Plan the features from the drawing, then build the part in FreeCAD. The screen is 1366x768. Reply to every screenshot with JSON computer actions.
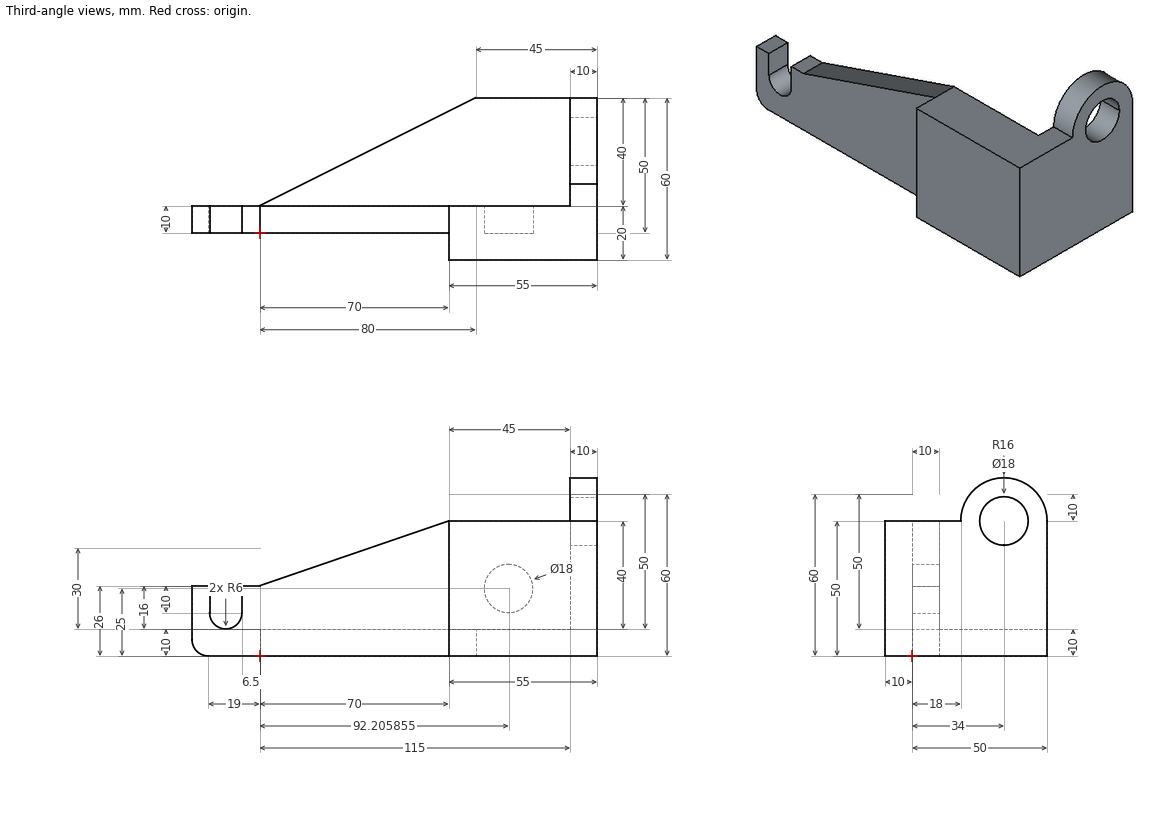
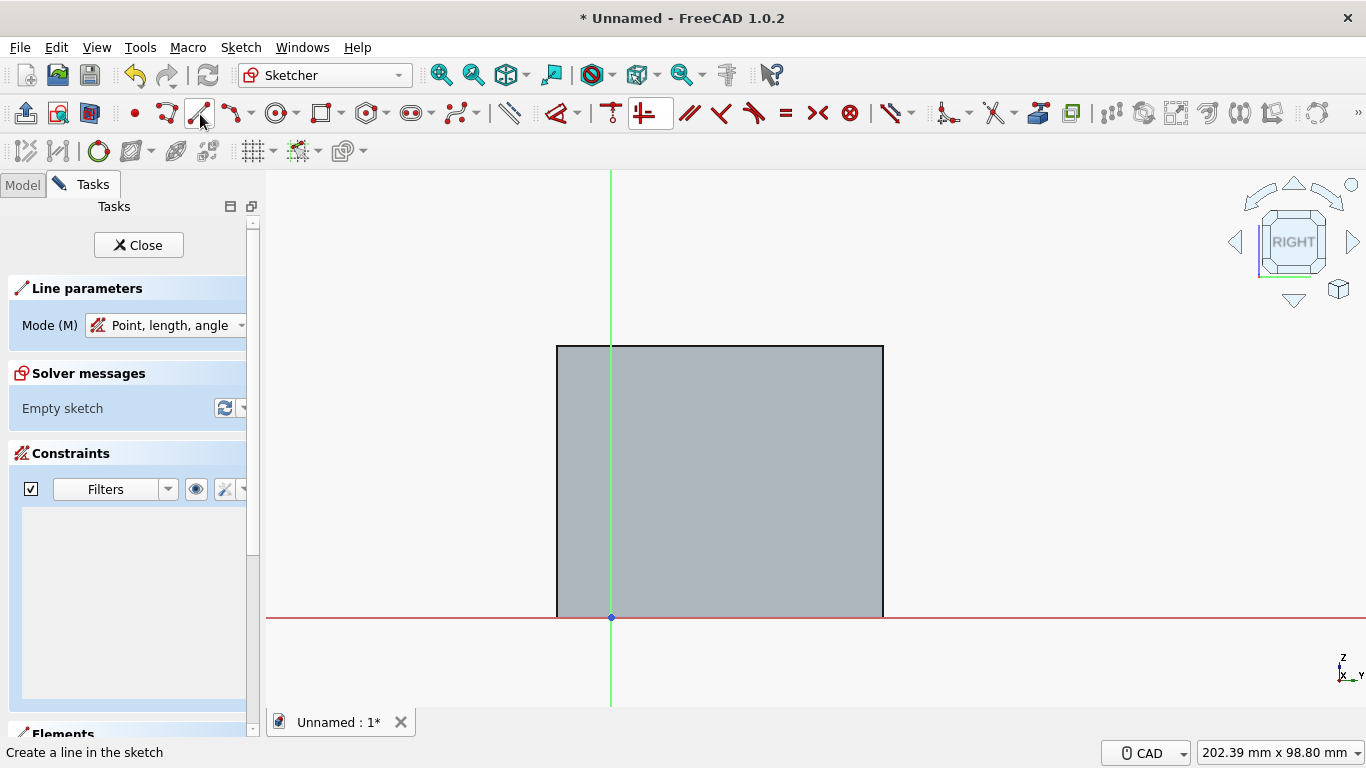
{"action": "left_click", "coordinate": [709, 346]}
{"action": "left_click", "coordinate": [883, 346]}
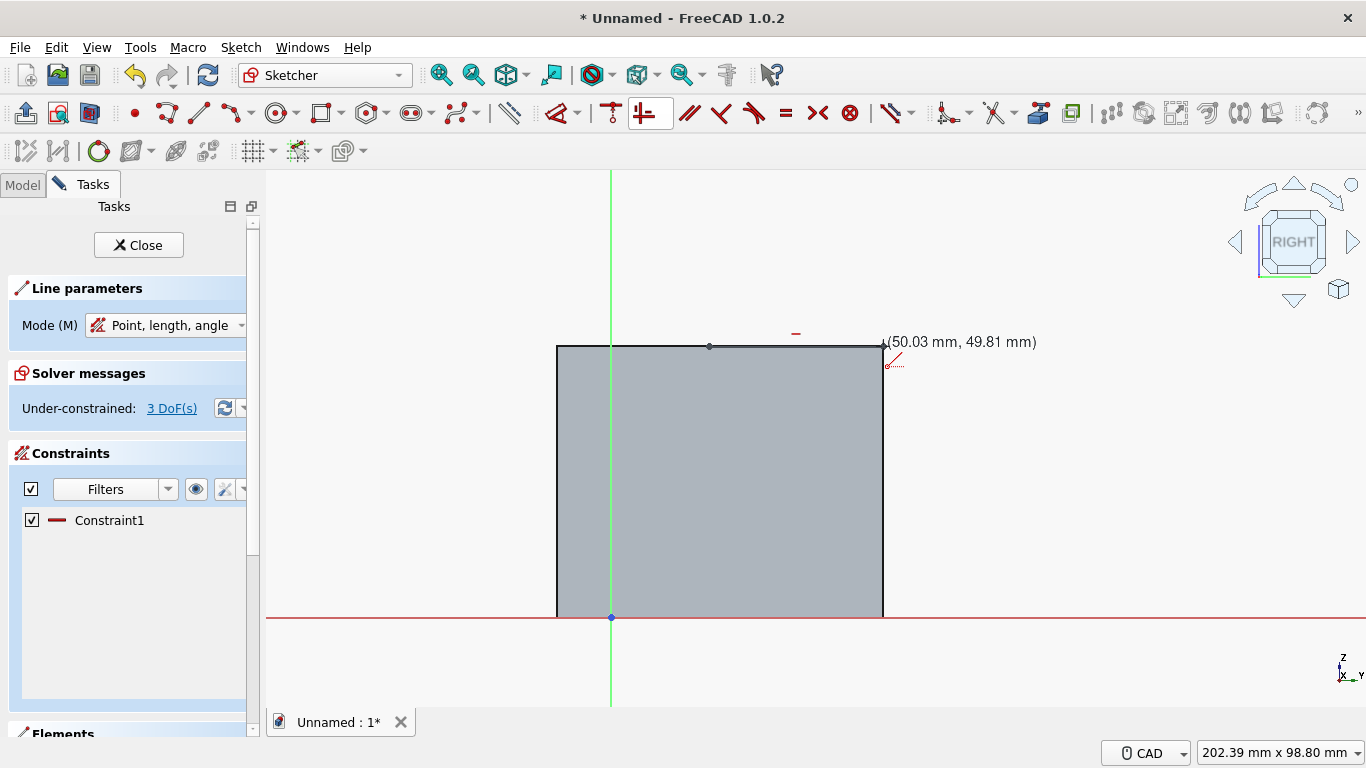
{"action": "left_click", "coordinate": [232, 114]}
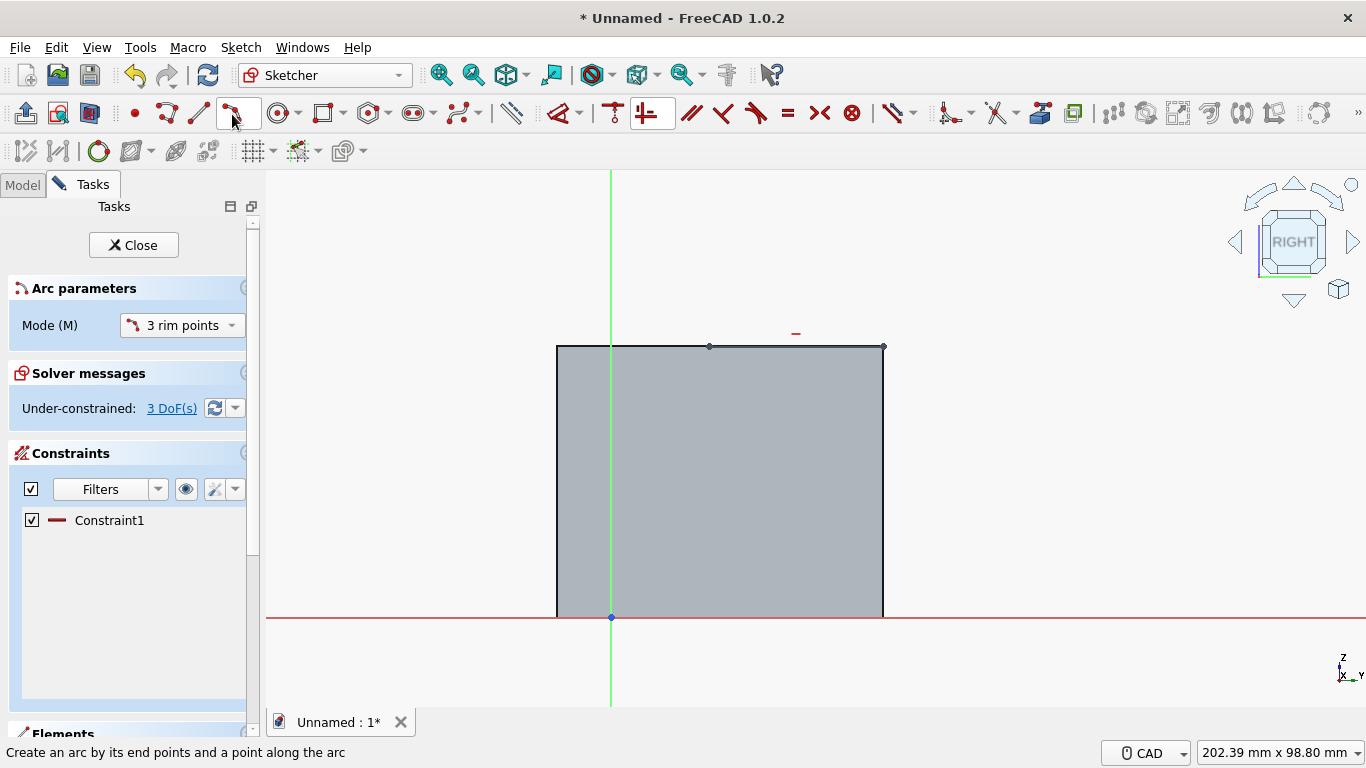
{"action": "left_click", "coordinate": [883, 347]}
{"action": "left_click", "coordinate": [709, 347]}
{"action": "left_click", "coordinate": [796, 259]}
{"action": "key", "text": "Escape"}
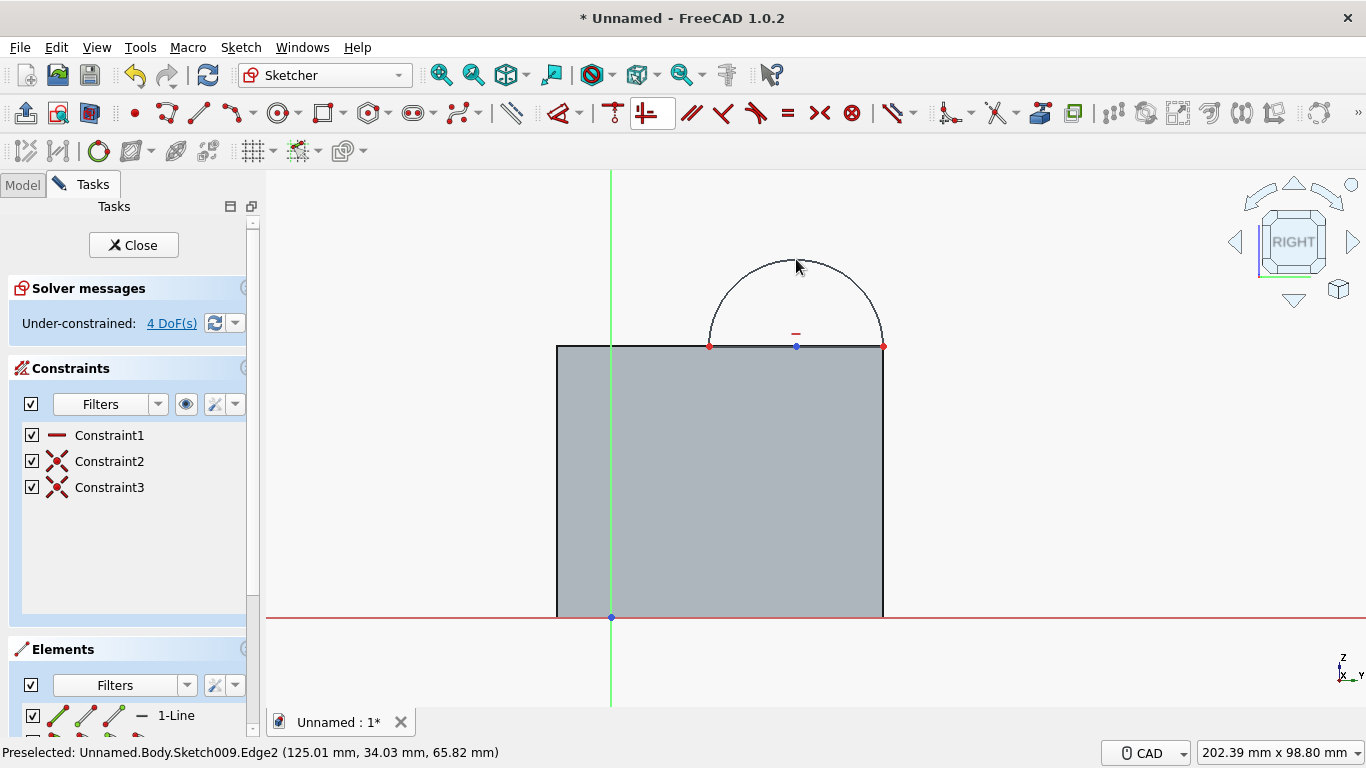
{"action": "left_click", "coordinate": [558, 114]}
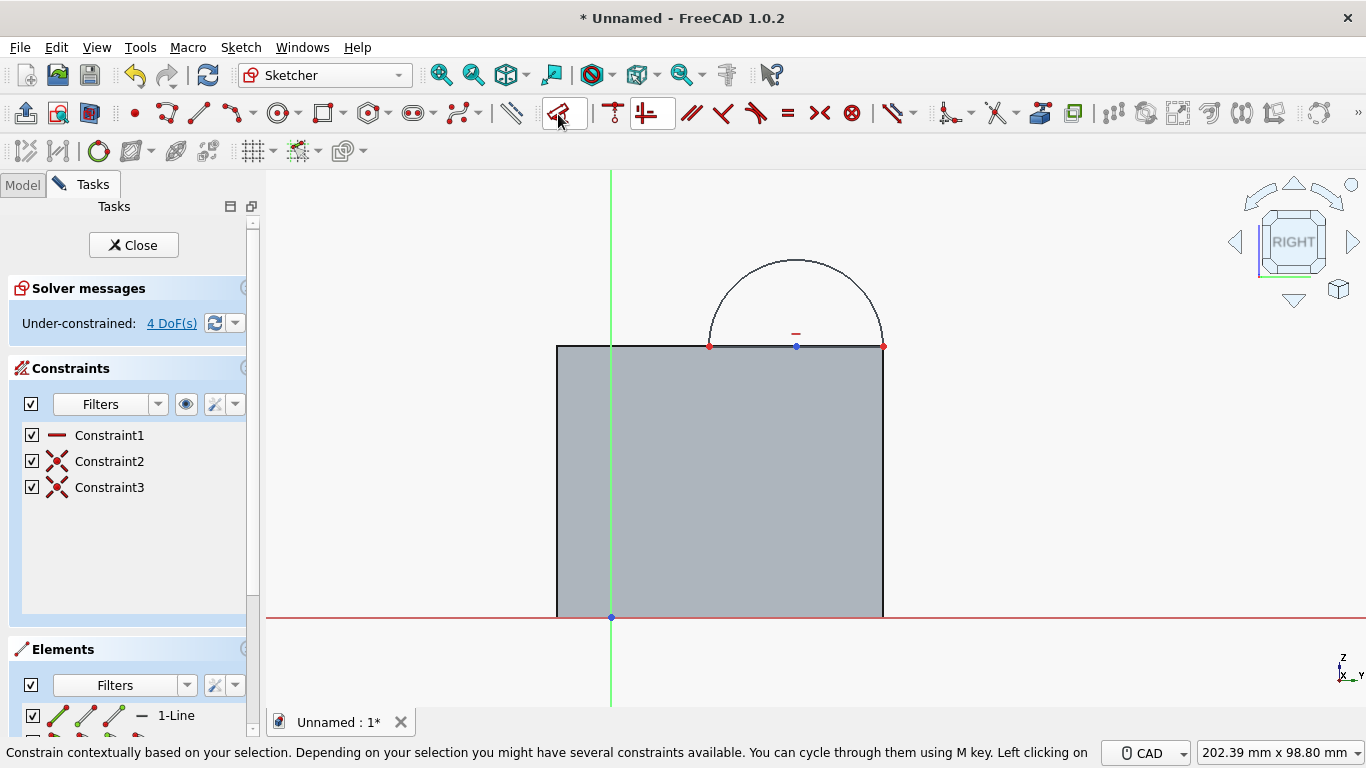
{"action": "left_click", "coordinate": [847, 277]}
{"action": "left_click", "coordinate": [866, 251]}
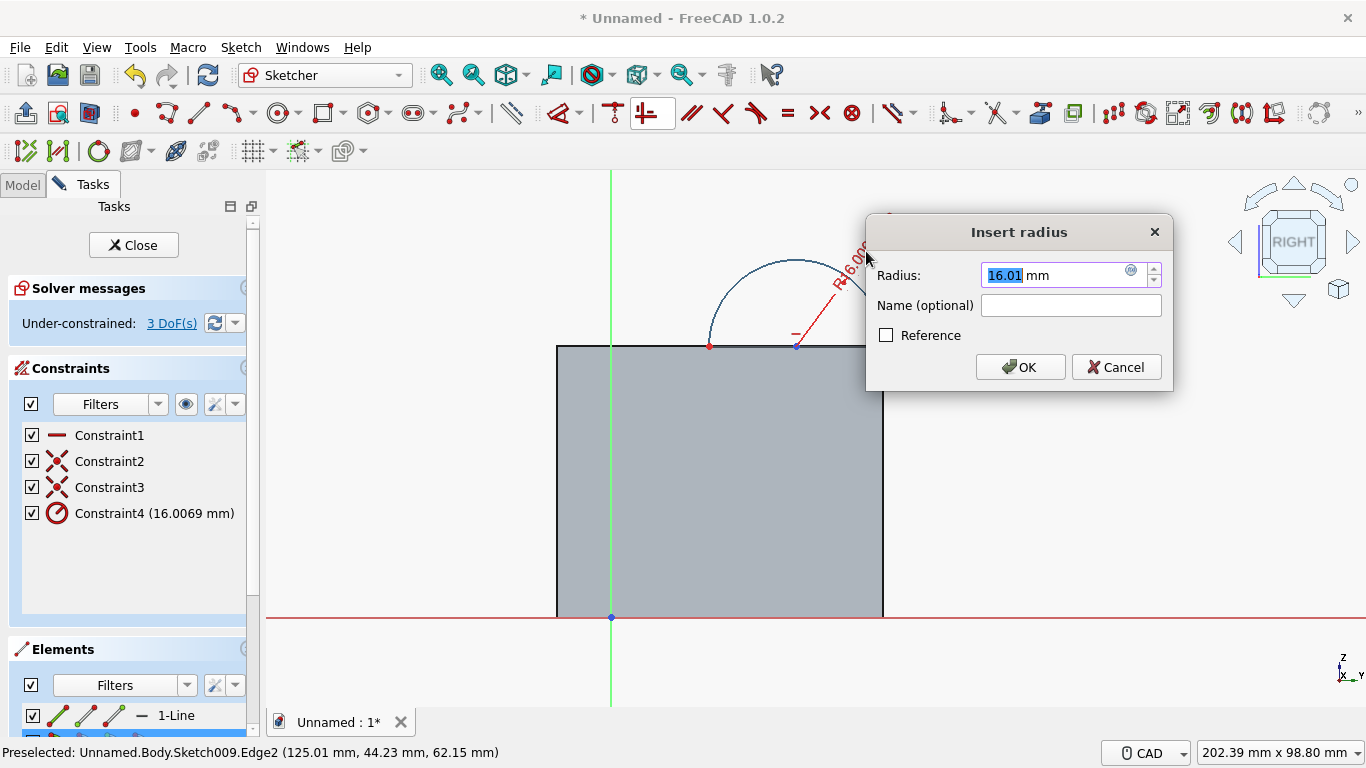
{"action": "type", "text": "16"}
{"action": "key", "text": "Return"}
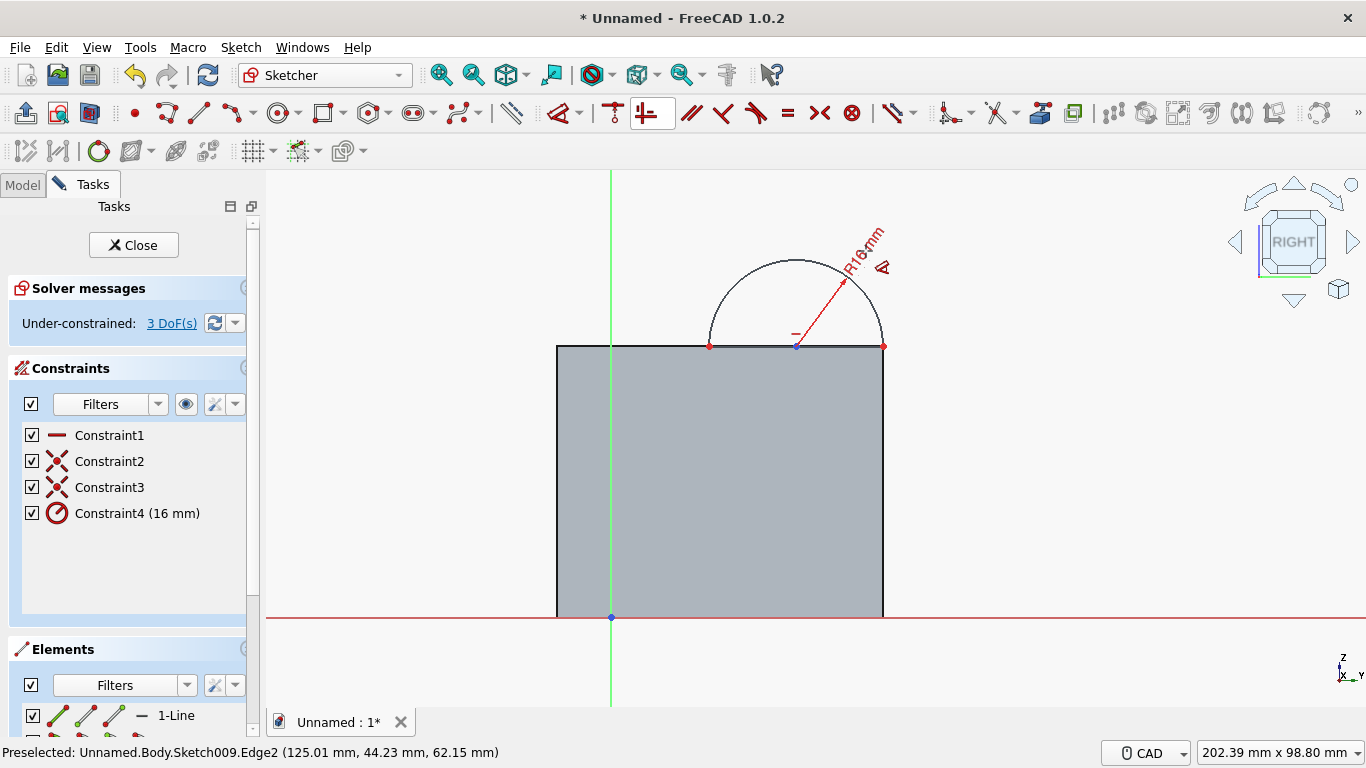
{"action": "left_click", "coordinate": [709, 347]}
{"action": "left_click", "coordinate": [660, 652]}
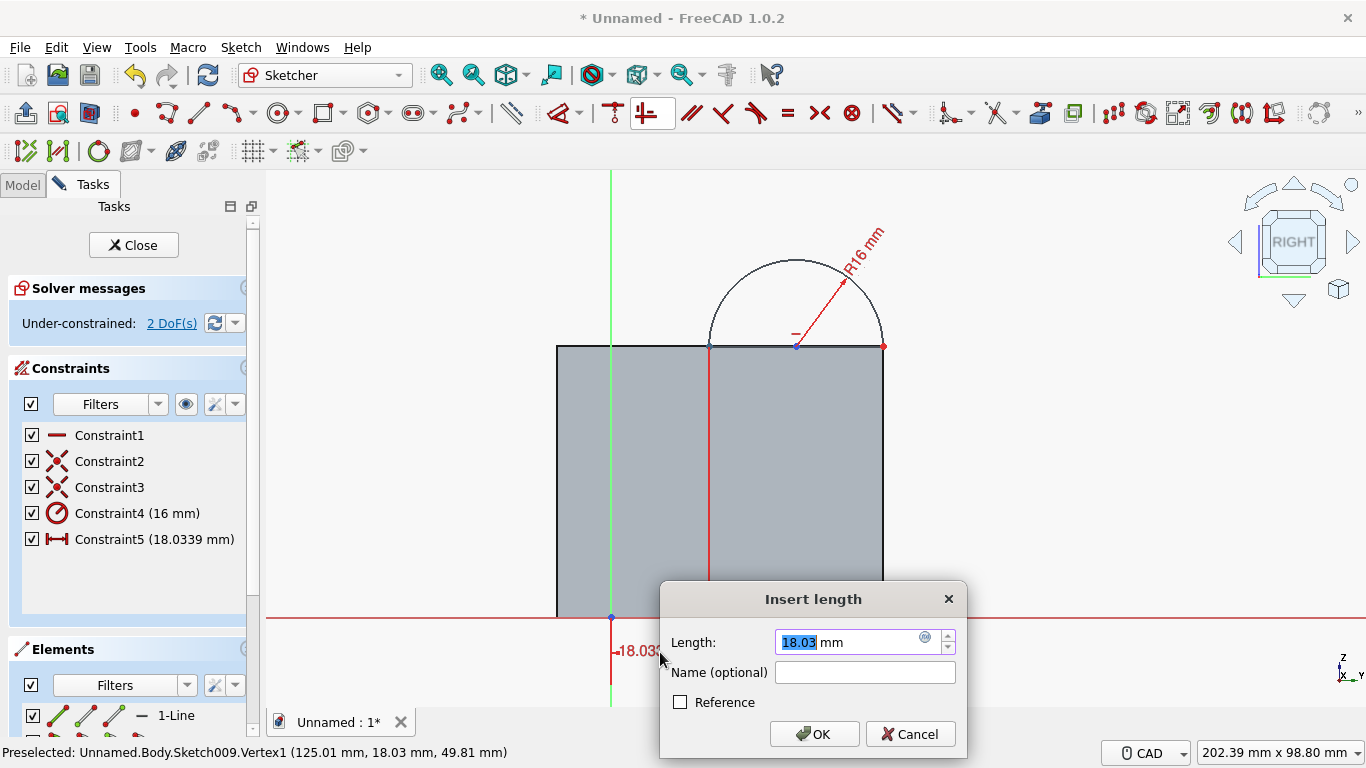
{"action": "type", "text": "18"}
{"action": "key", "text": "Return"}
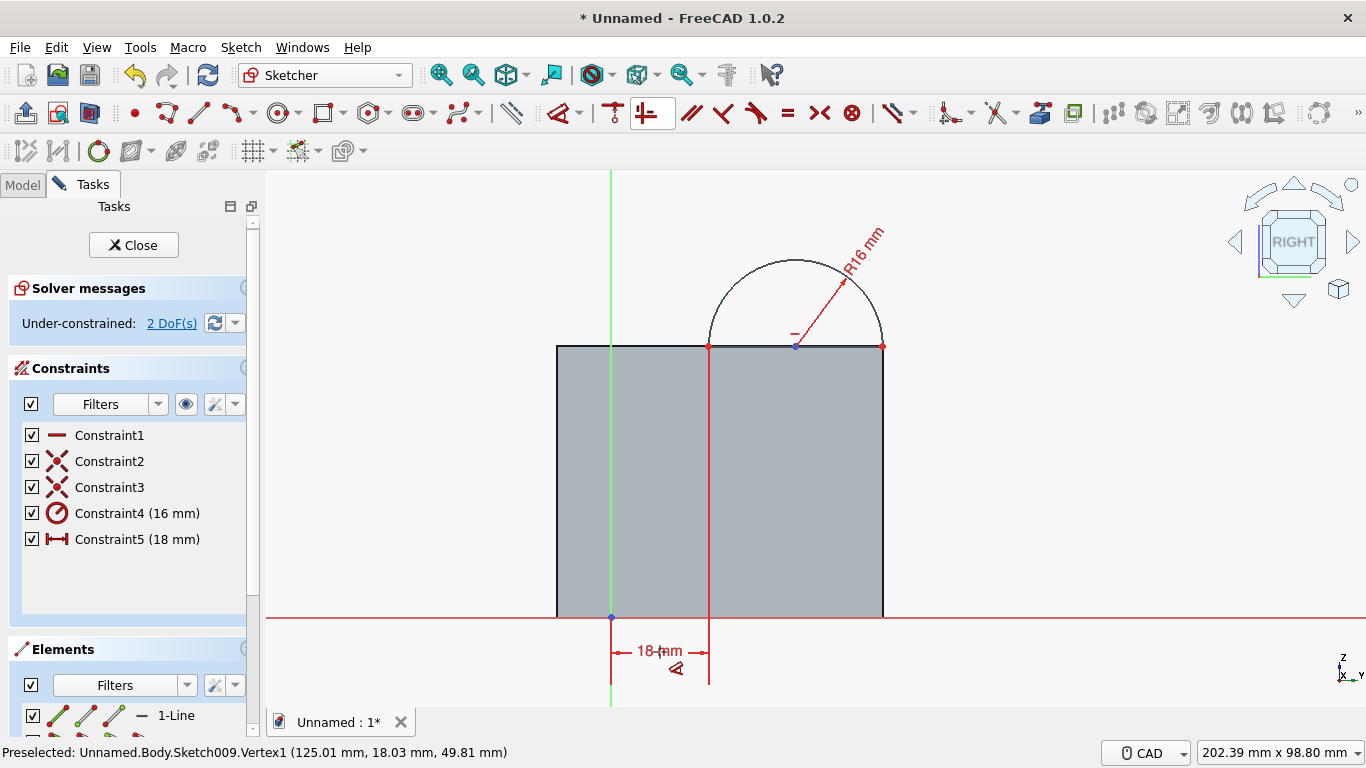
{"action": "left_click", "coordinate": [709, 347]}
{"action": "left_click", "coordinate": [577, 482]}